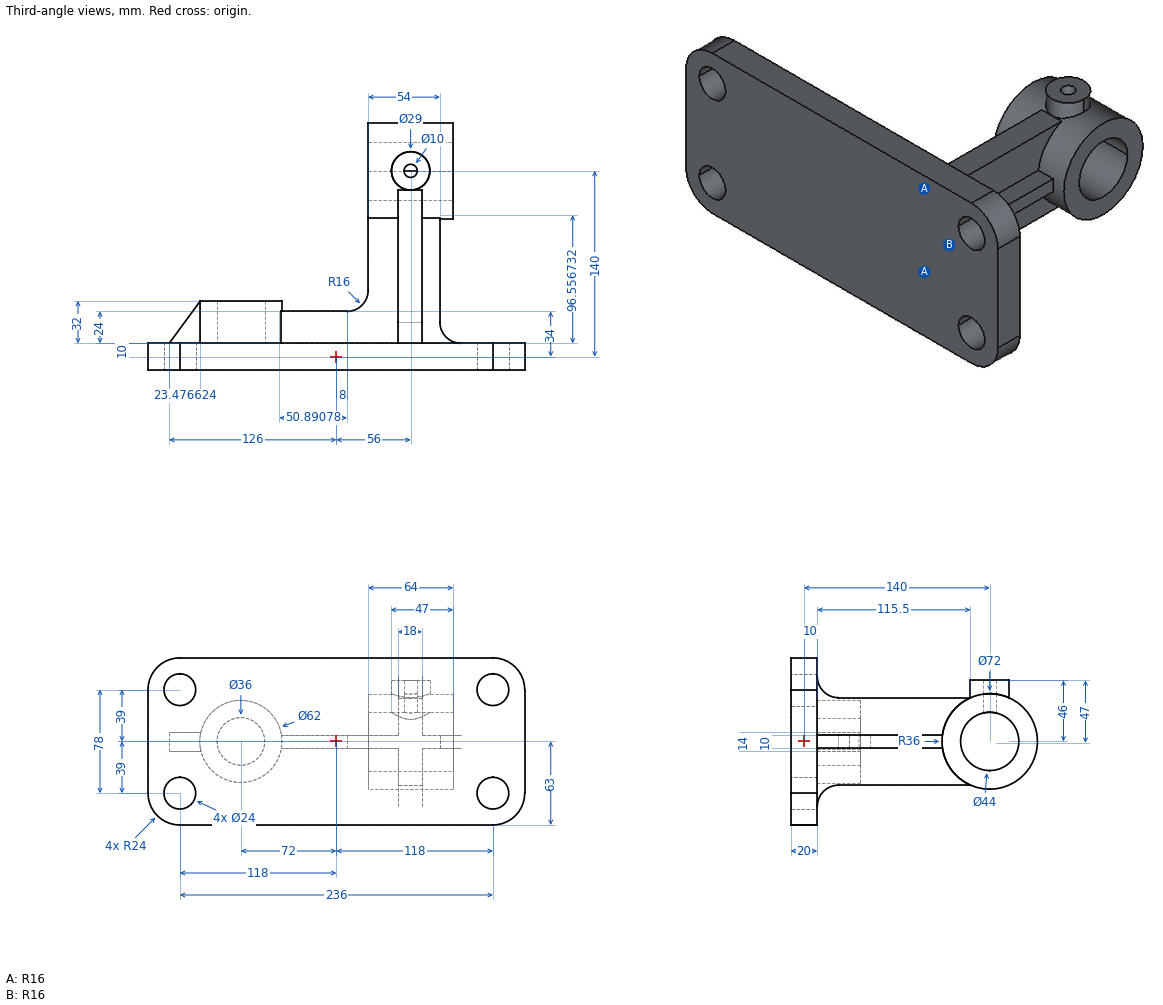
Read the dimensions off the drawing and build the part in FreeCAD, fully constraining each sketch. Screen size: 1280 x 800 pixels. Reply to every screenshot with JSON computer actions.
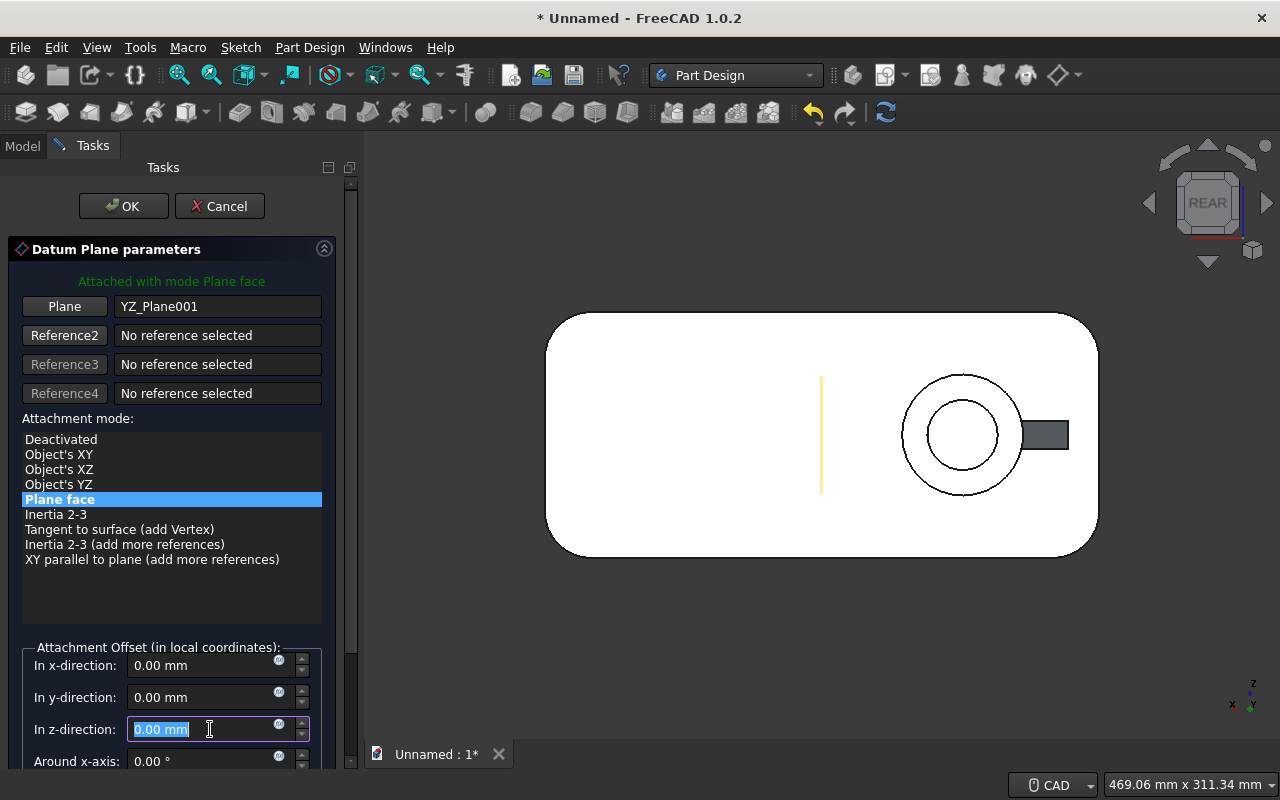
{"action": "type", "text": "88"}
{"action": "key", "text": "Tab"}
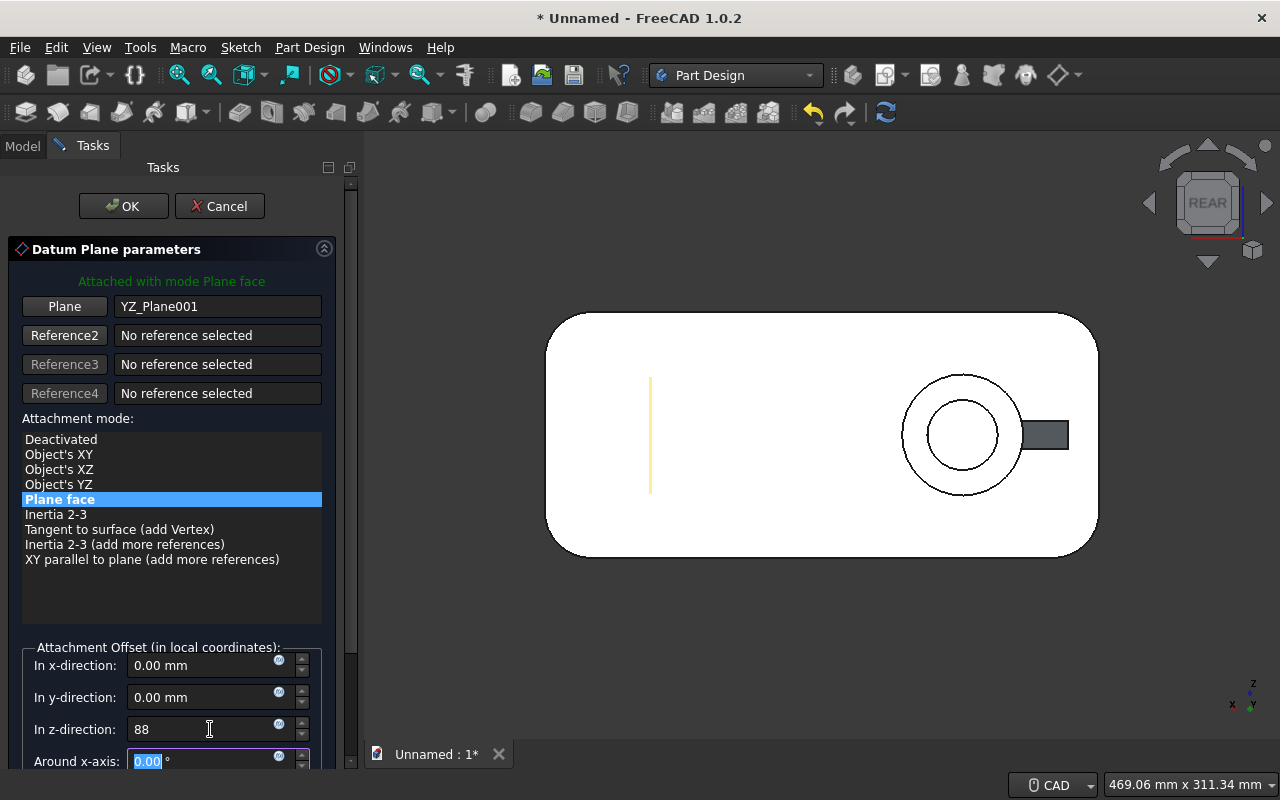
{"action": "left_click", "coordinate": [124, 206]}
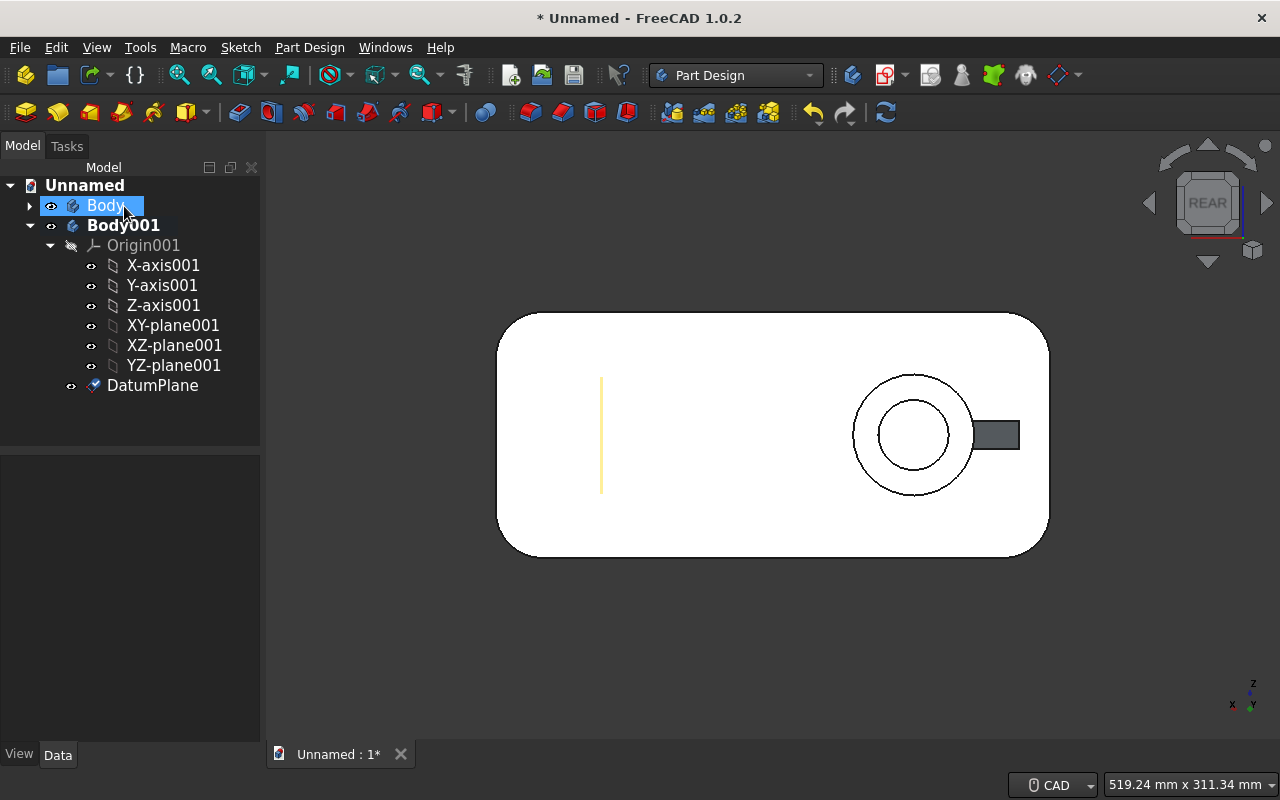
{"action": "left_click", "coordinate": [116, 386]}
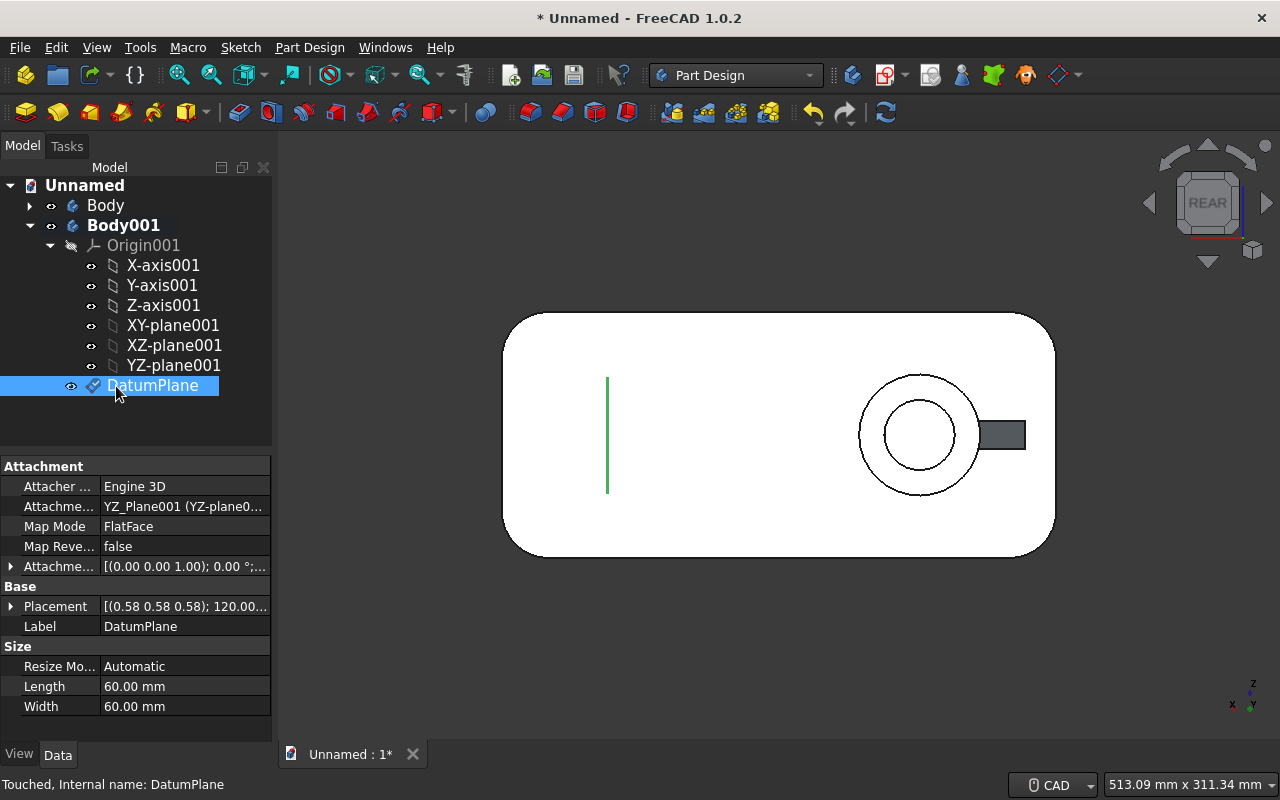
{"action": "left_click", "coordinate": [886, 76]}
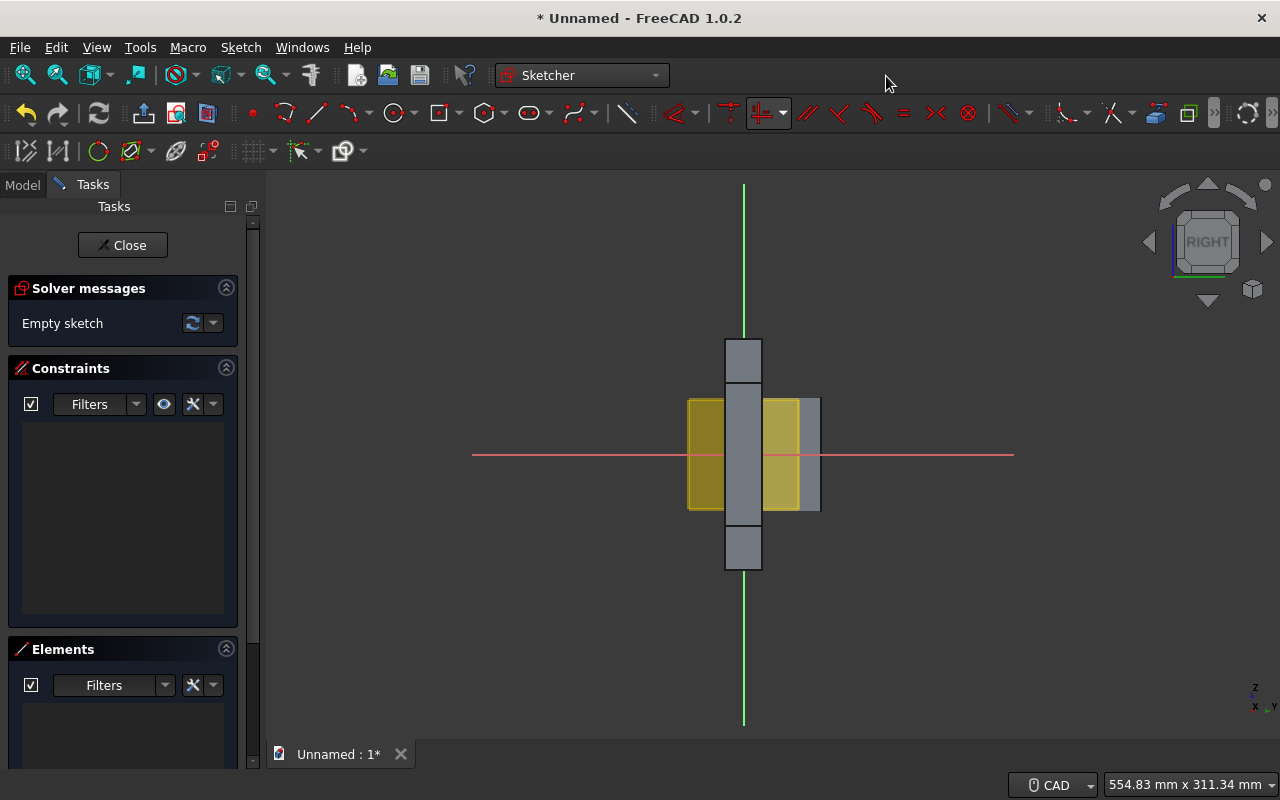
{"action": "scroll", "coordinate": [1115, 455], "scroll_direction": "up", "scroll_amount": 3}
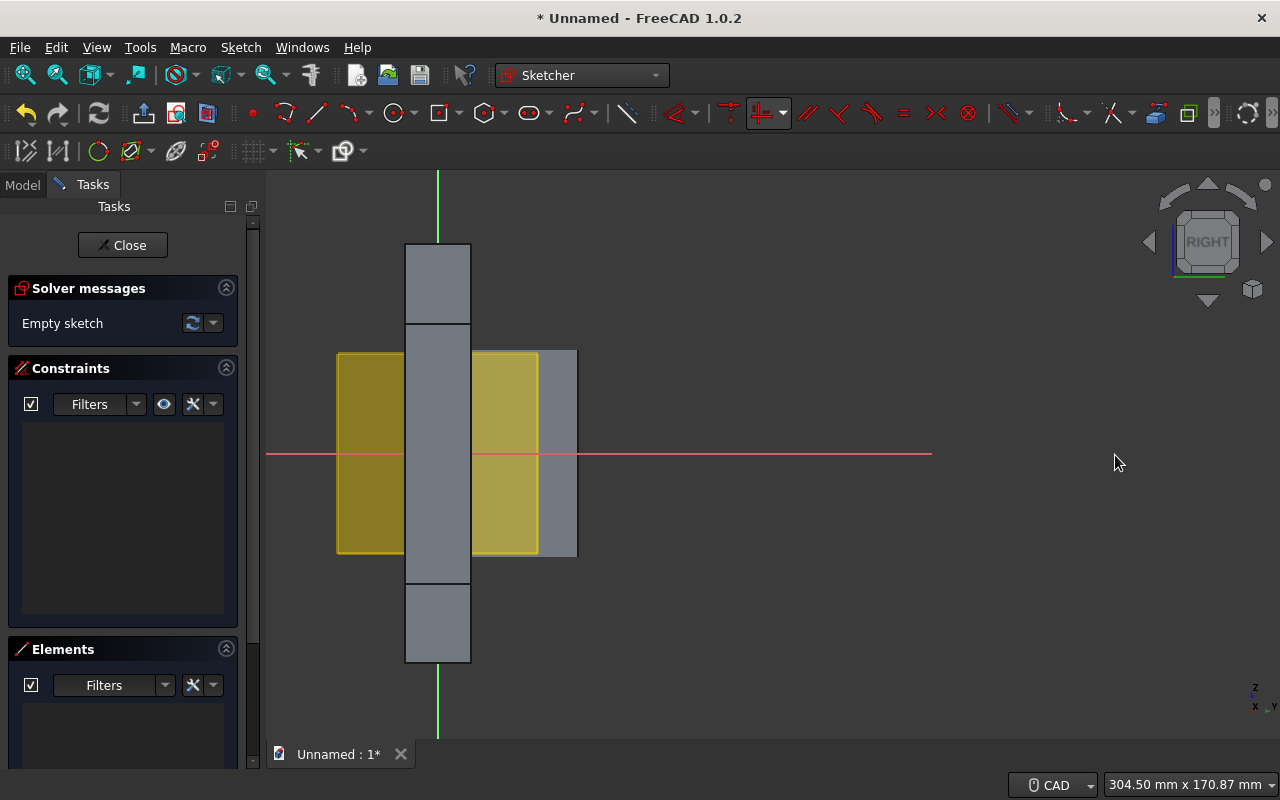
{"action": "left_click", "coordinate": [394, 114]}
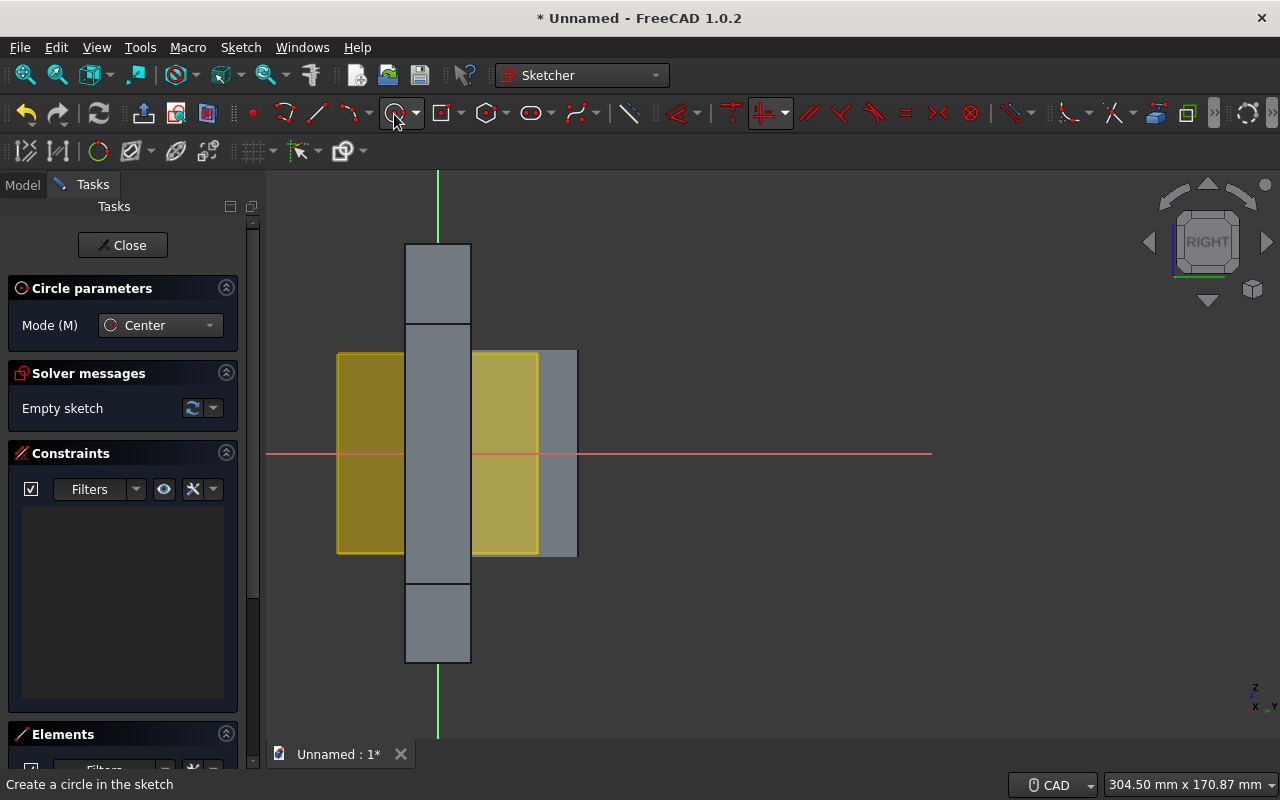
{"action": "left_click", "coordinate": [904, 454]}
{"action": "mouse_move", "coordinate": [989, 369]}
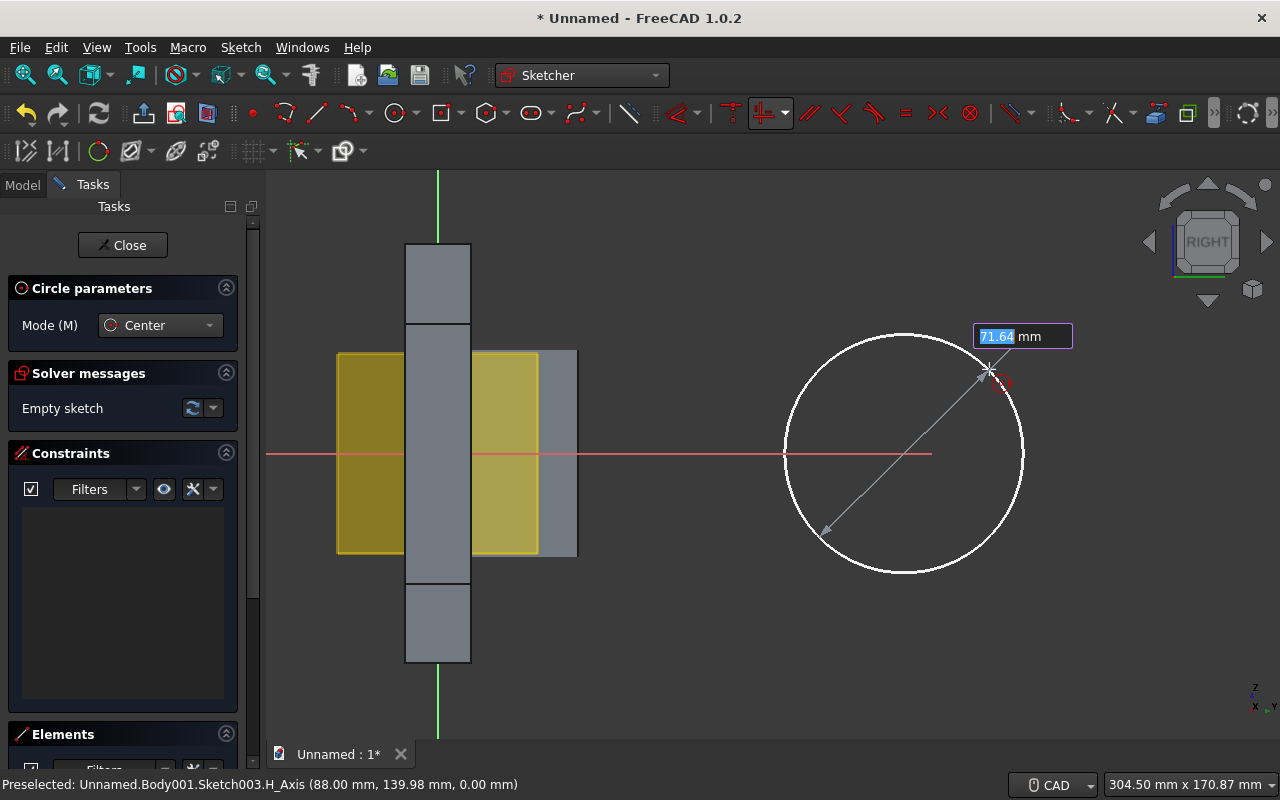
{"action": "type", "text": "72"}
{"action": "key", "text": "Return"}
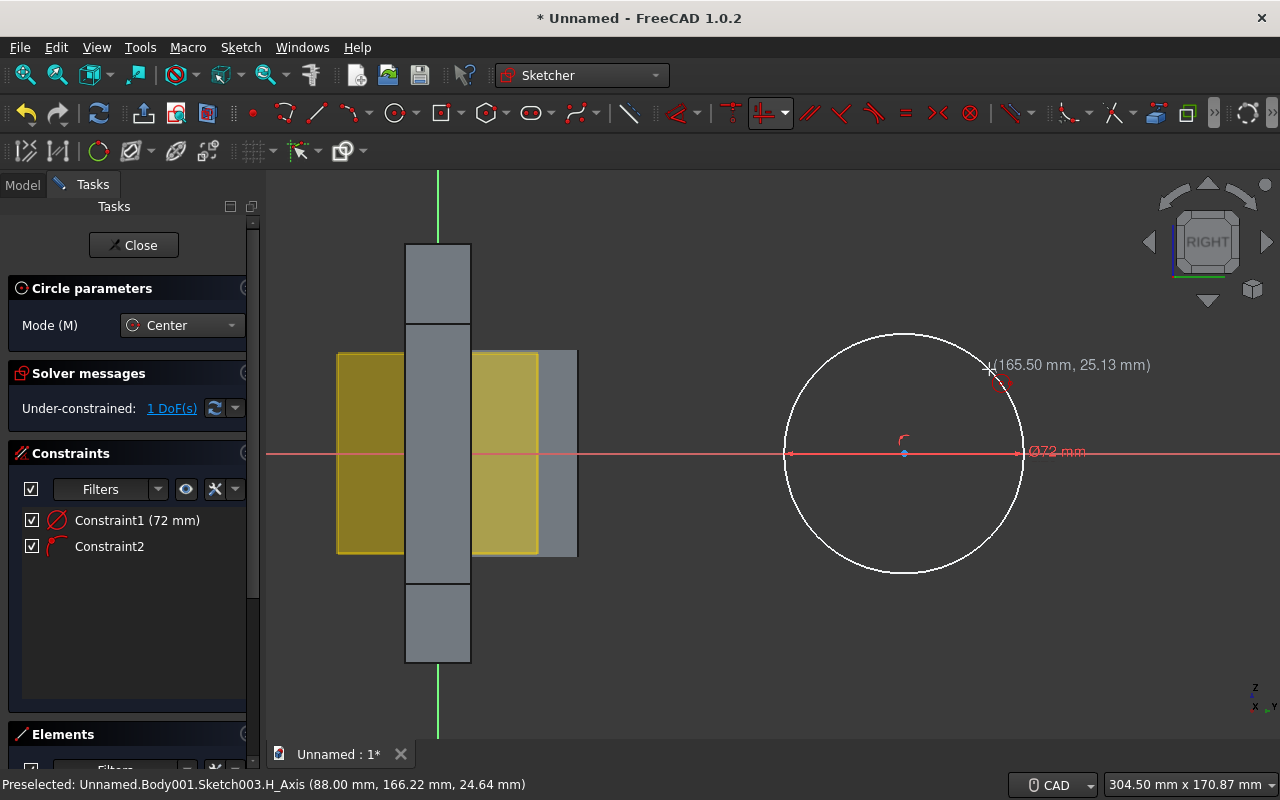
{"action": "left_click", "coordinate": [904, 454]}
{"action": "mouse_move", "coordinate": [956, 402]}